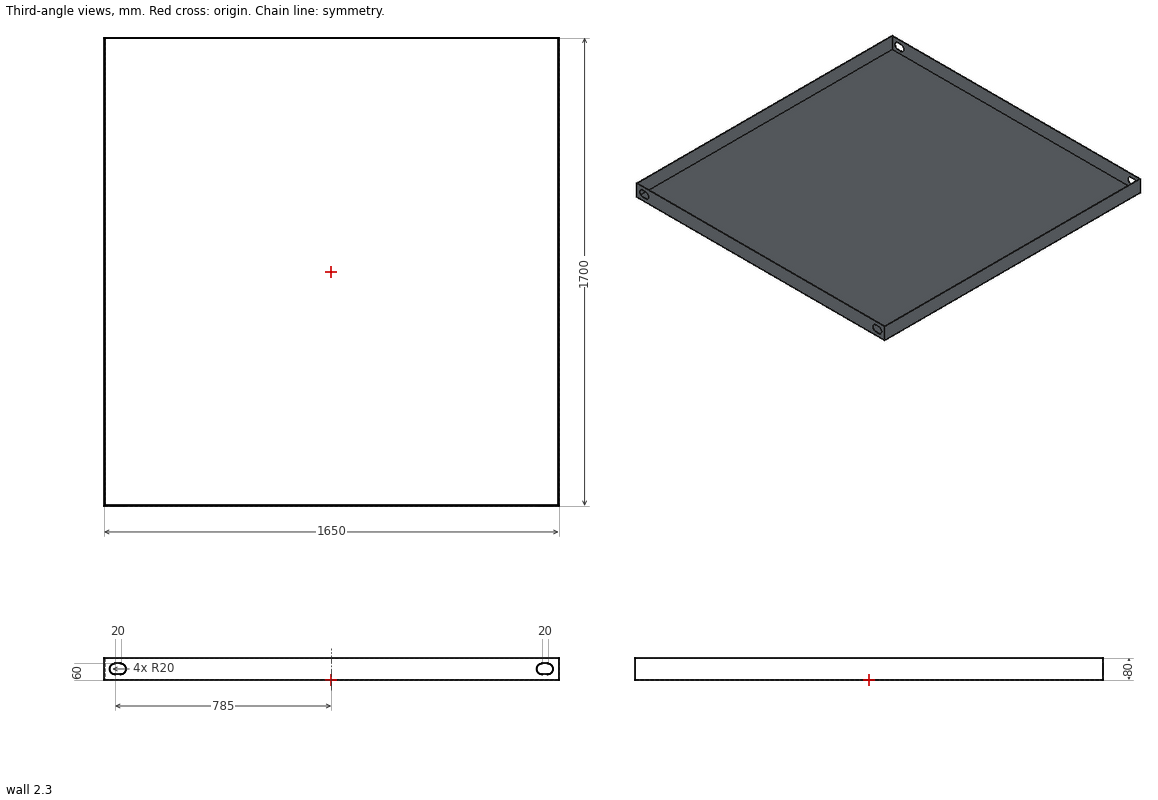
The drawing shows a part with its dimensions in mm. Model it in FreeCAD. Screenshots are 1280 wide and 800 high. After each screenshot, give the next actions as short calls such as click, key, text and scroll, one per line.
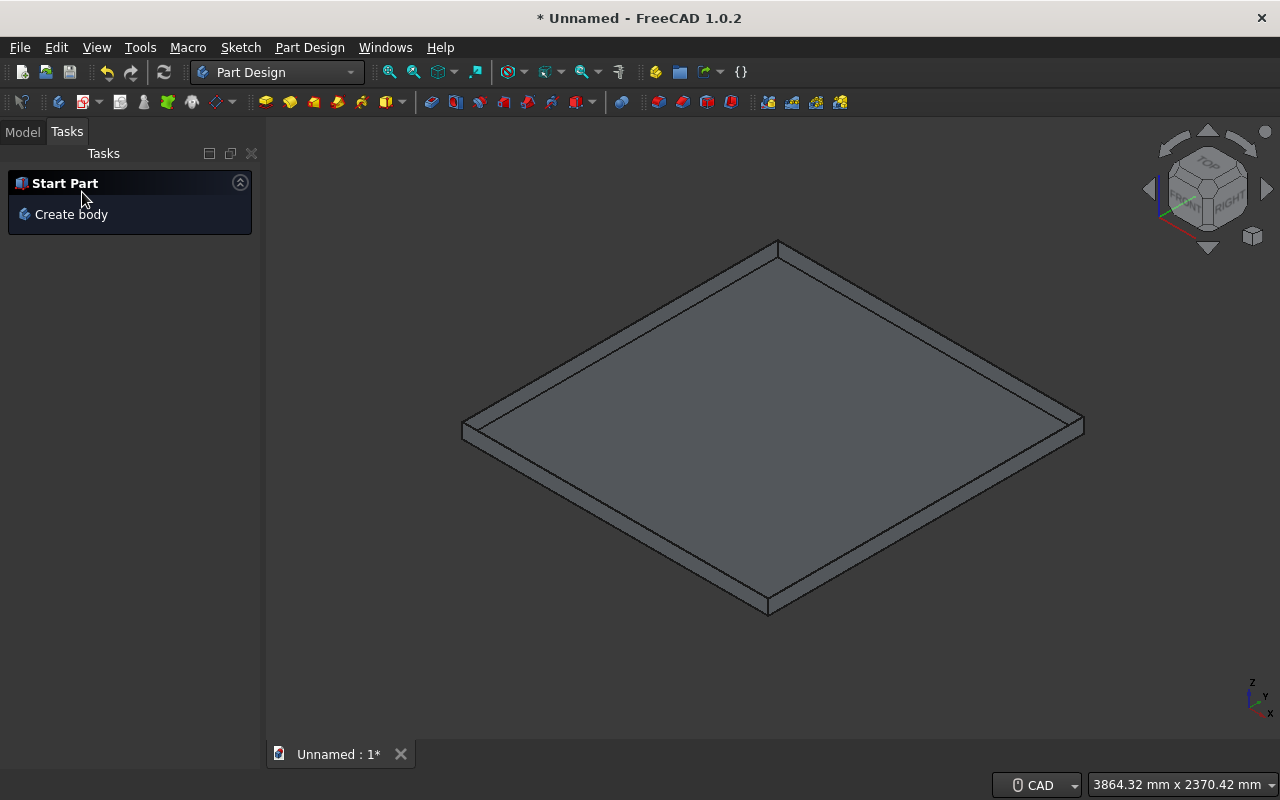
key(1)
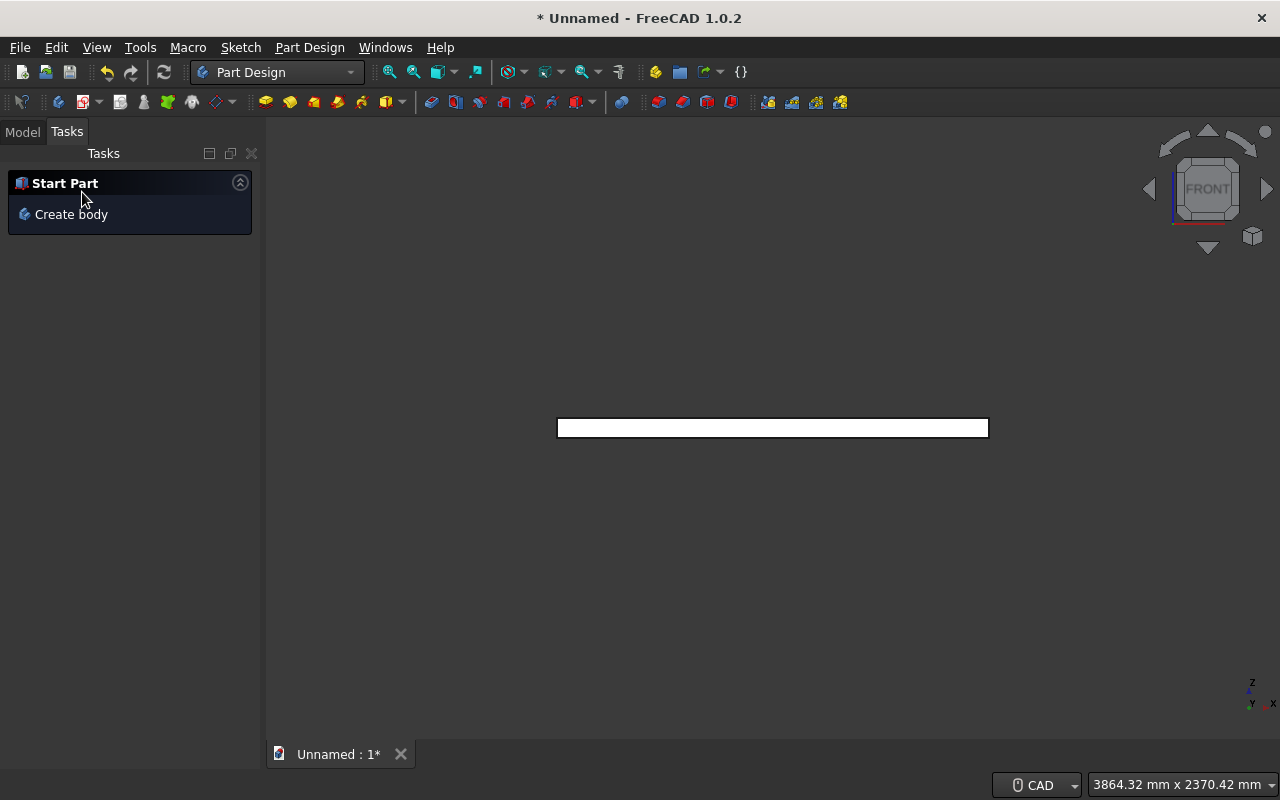
key(v)
key(f)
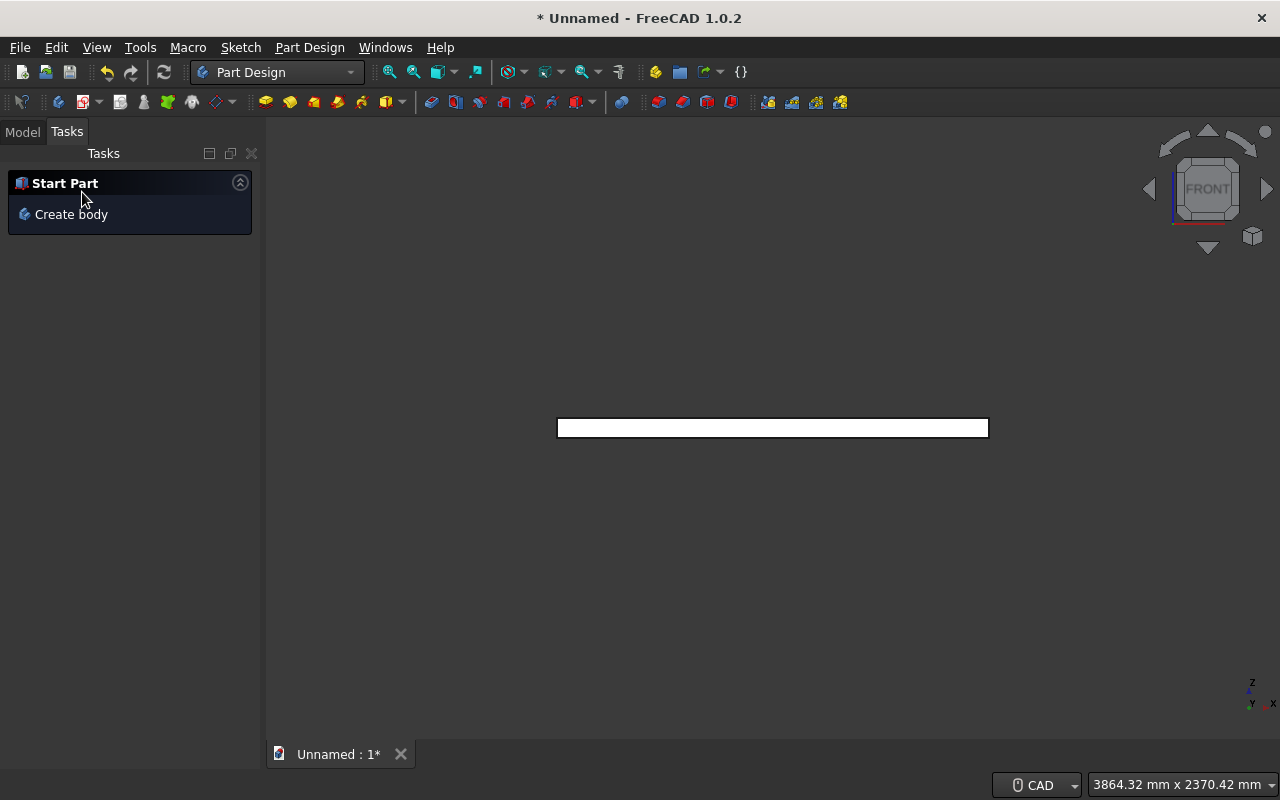
click(959, 427)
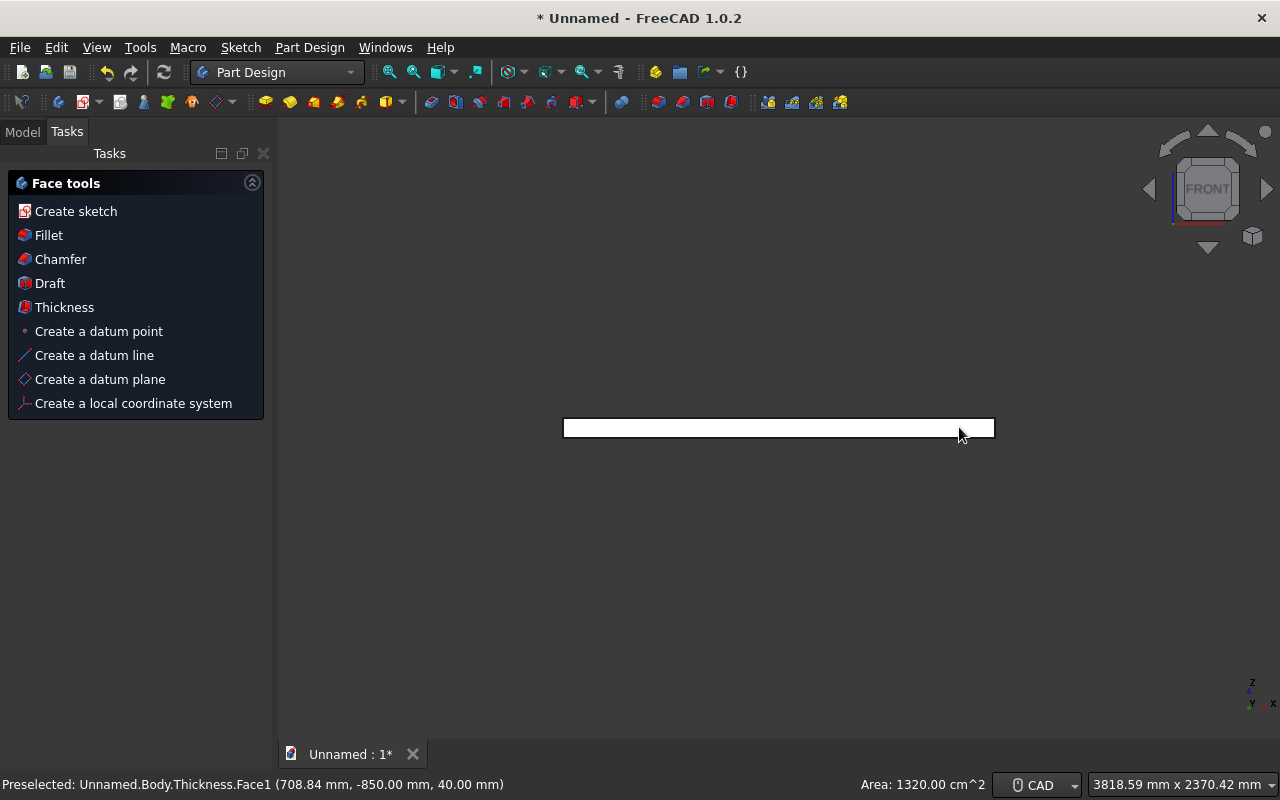
click(84, 102)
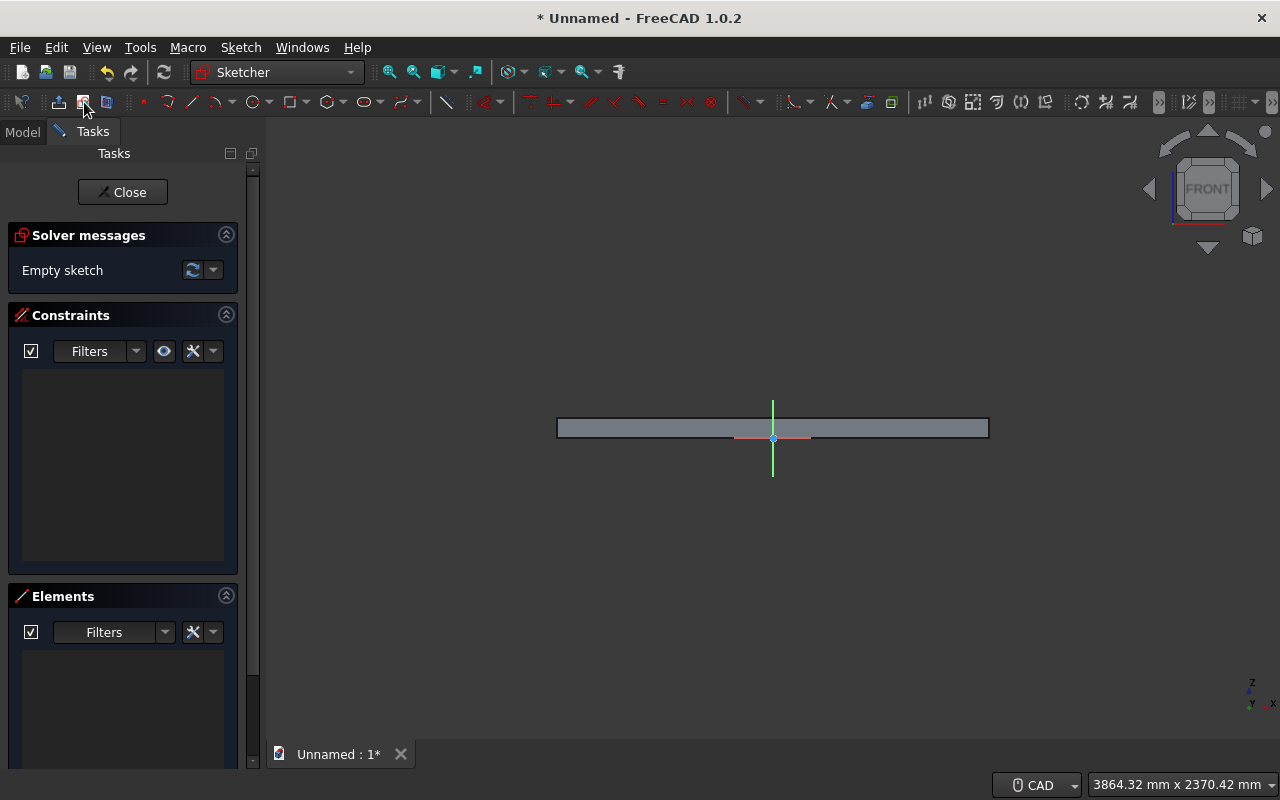
scroll(912, 436, up, 2)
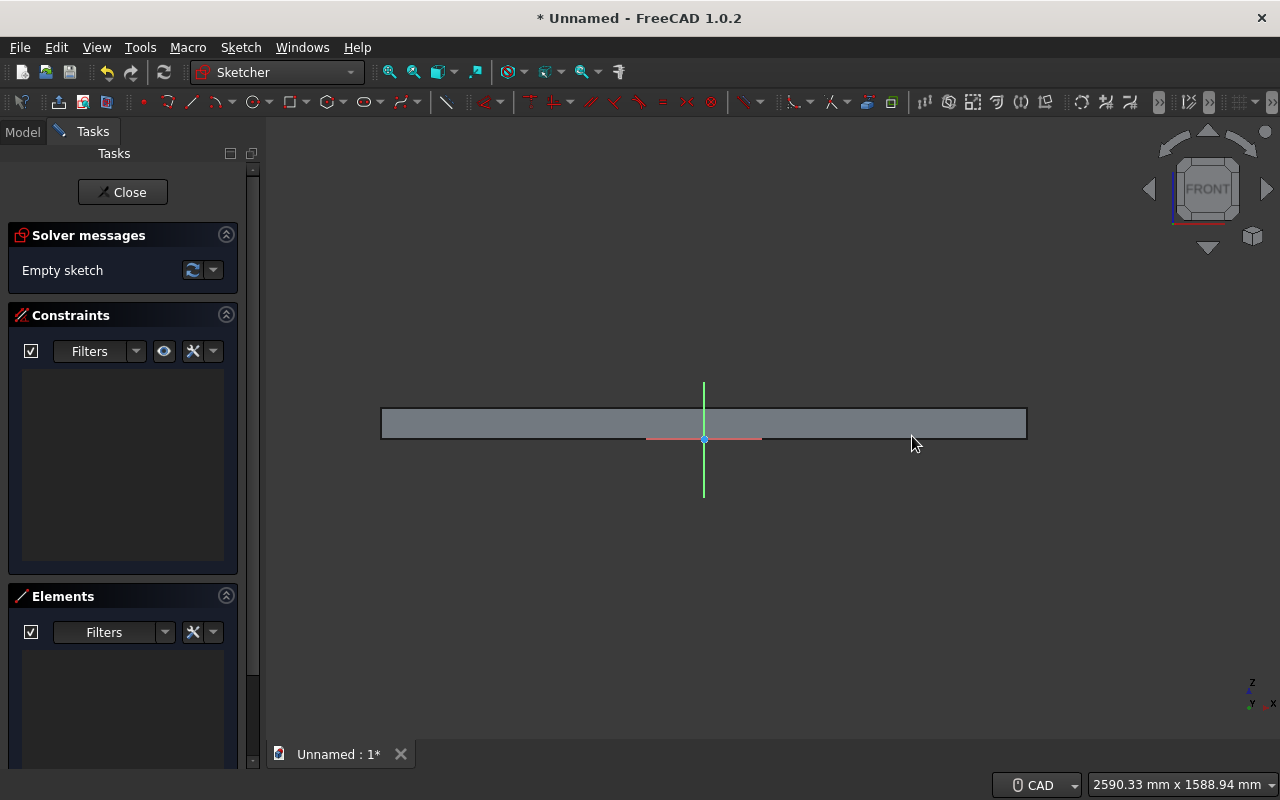
key(g)
key(s)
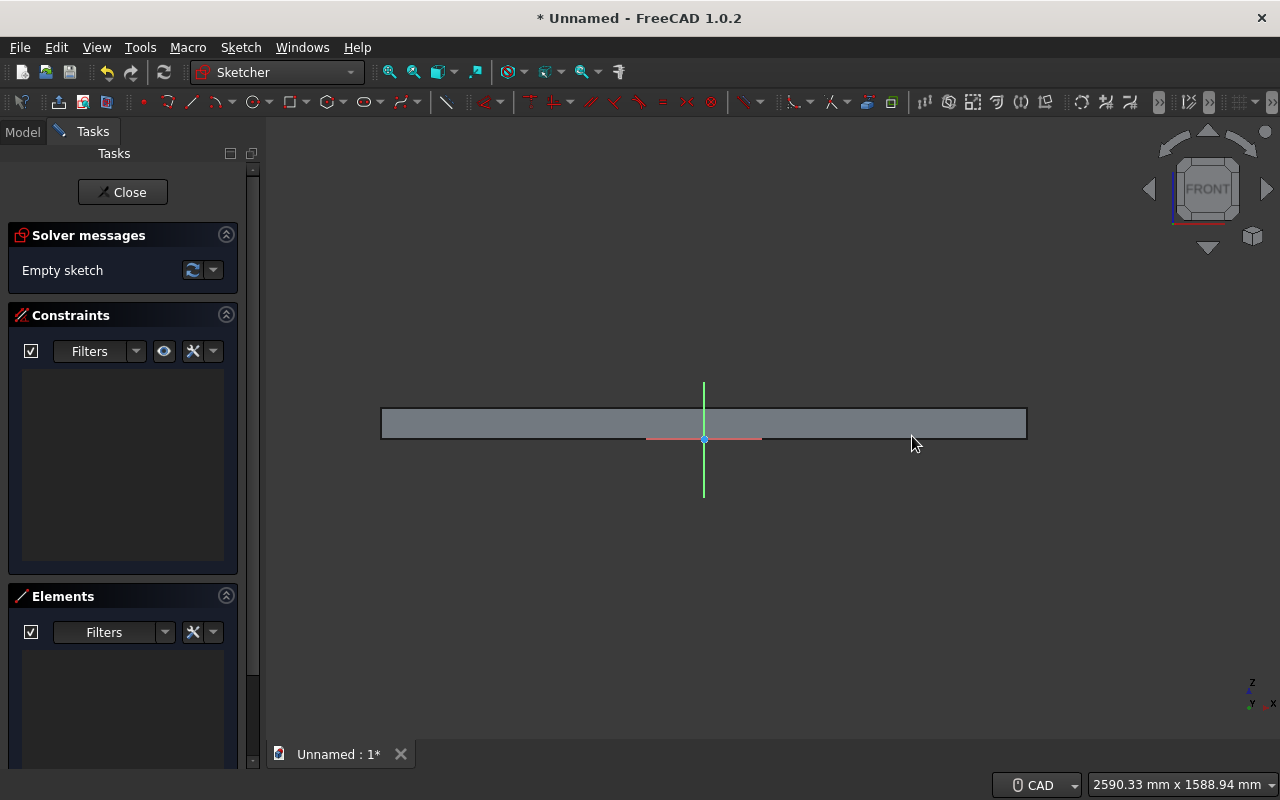
scroll(397, 424, up, 6)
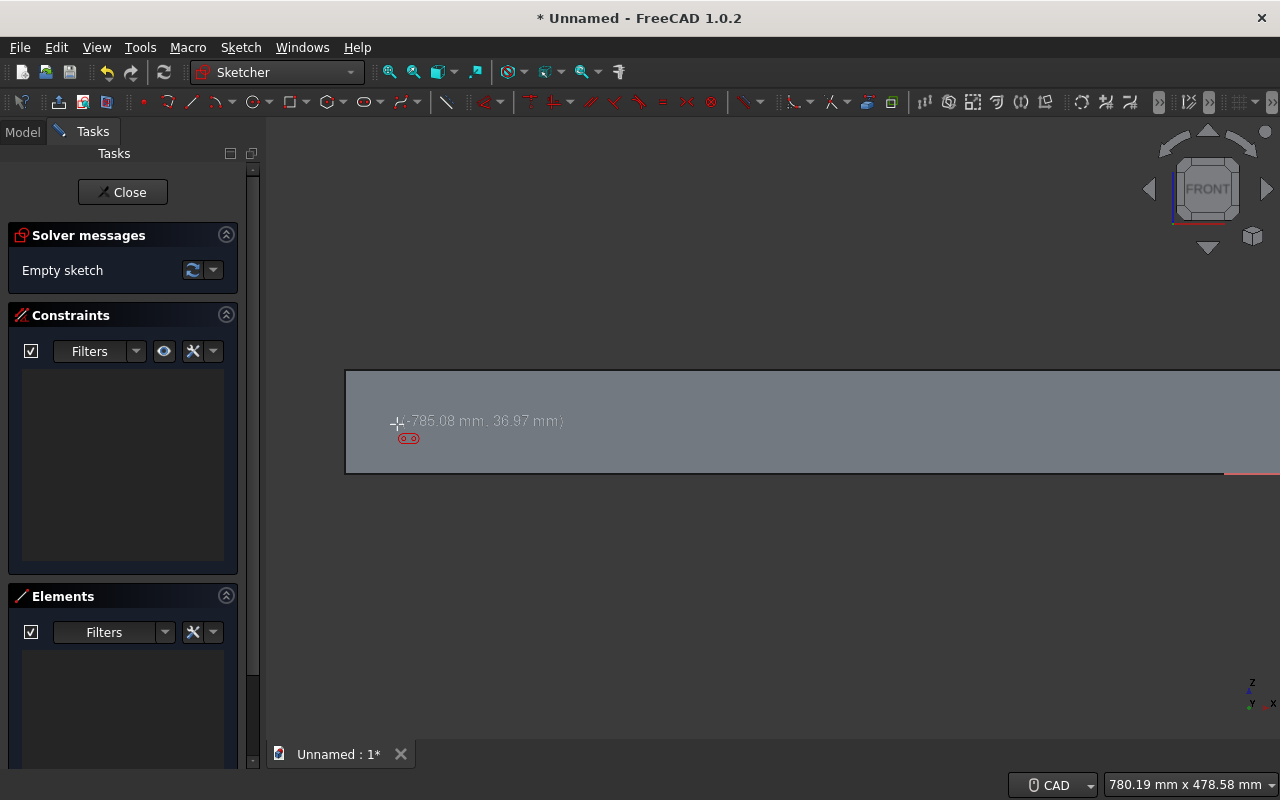
click(397, 422)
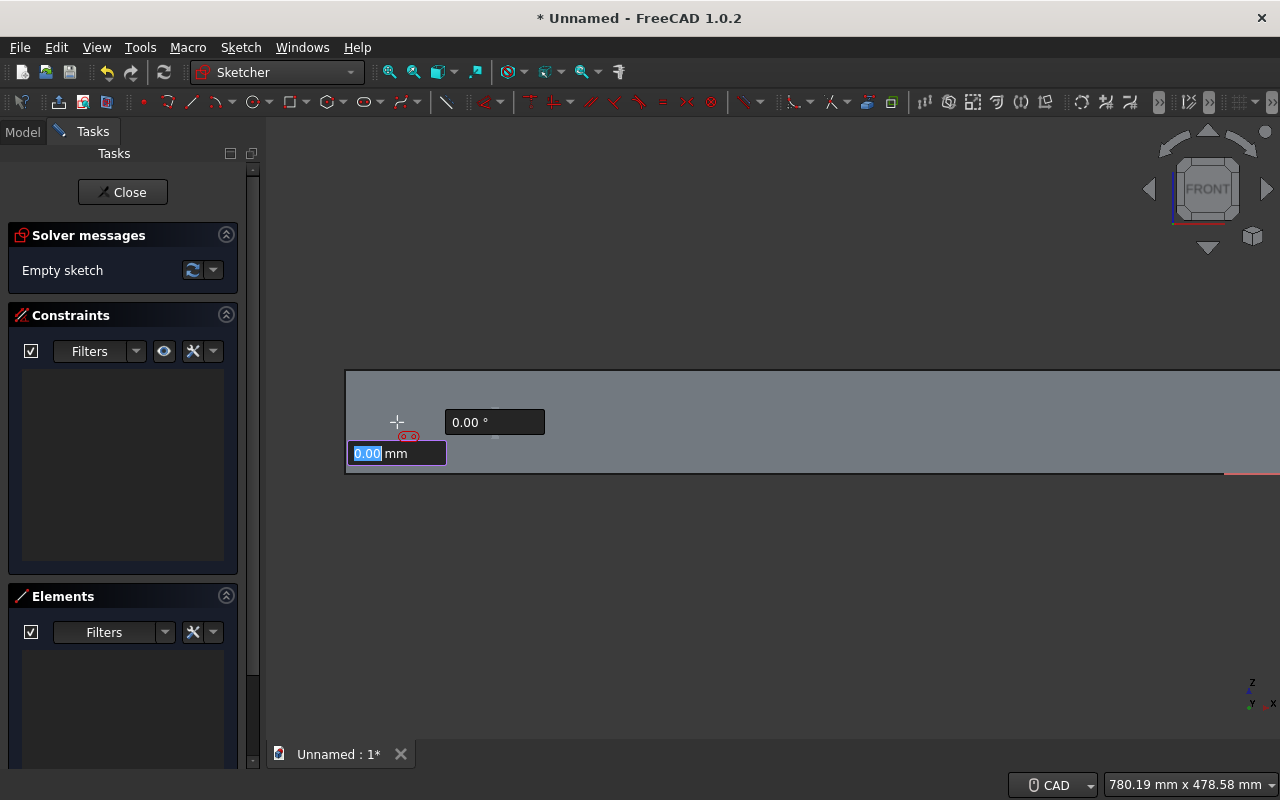
click(423, 422)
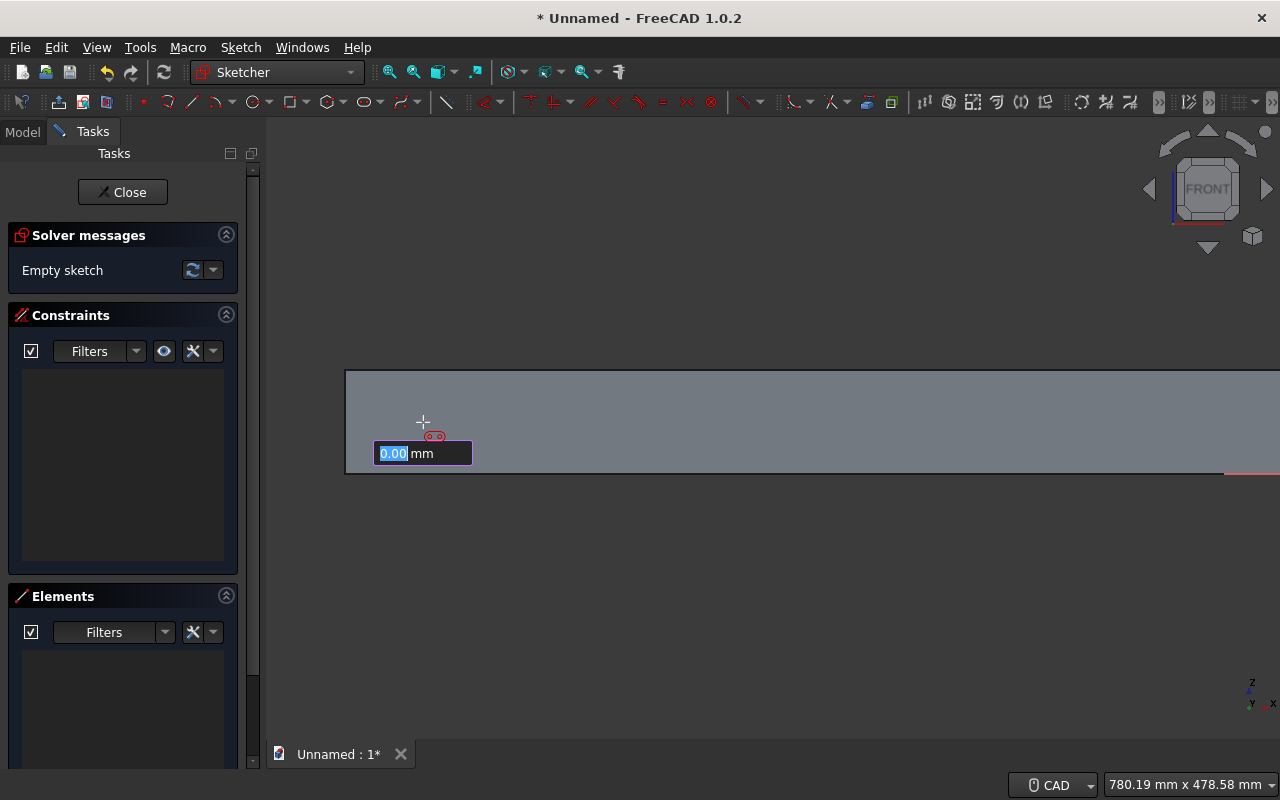
click(410, 396)